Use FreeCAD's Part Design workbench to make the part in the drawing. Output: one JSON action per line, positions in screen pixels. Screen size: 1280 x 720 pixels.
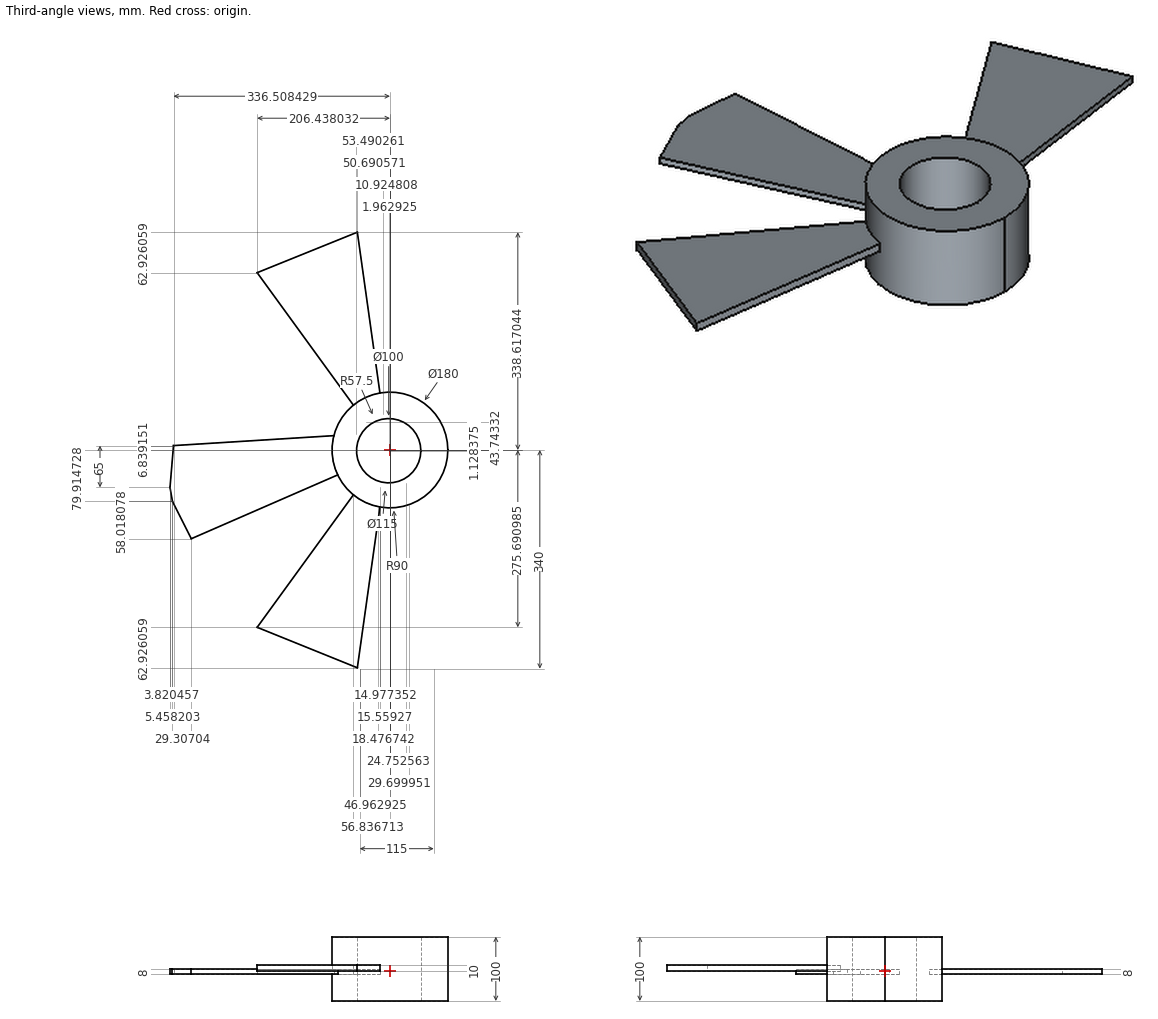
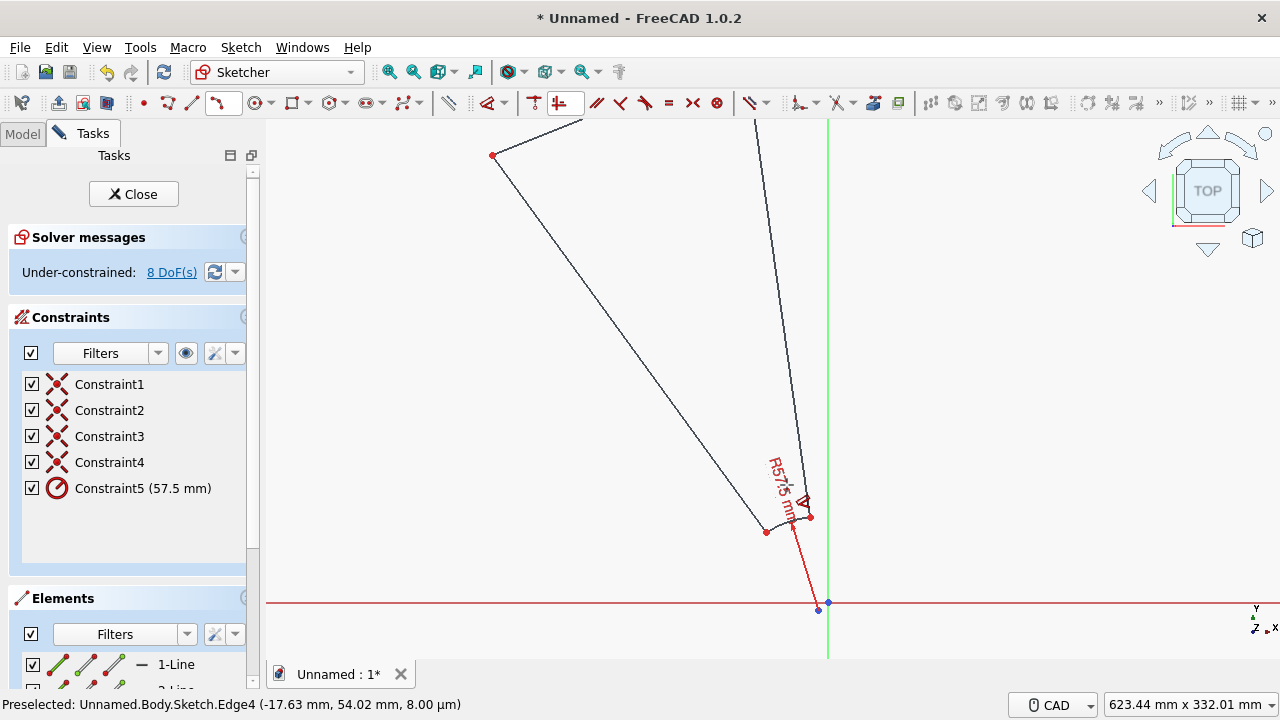
{"action": "left_click", "coordinate": [766, 533]}
{"action": "left_click", "coordinate": [862, 568]}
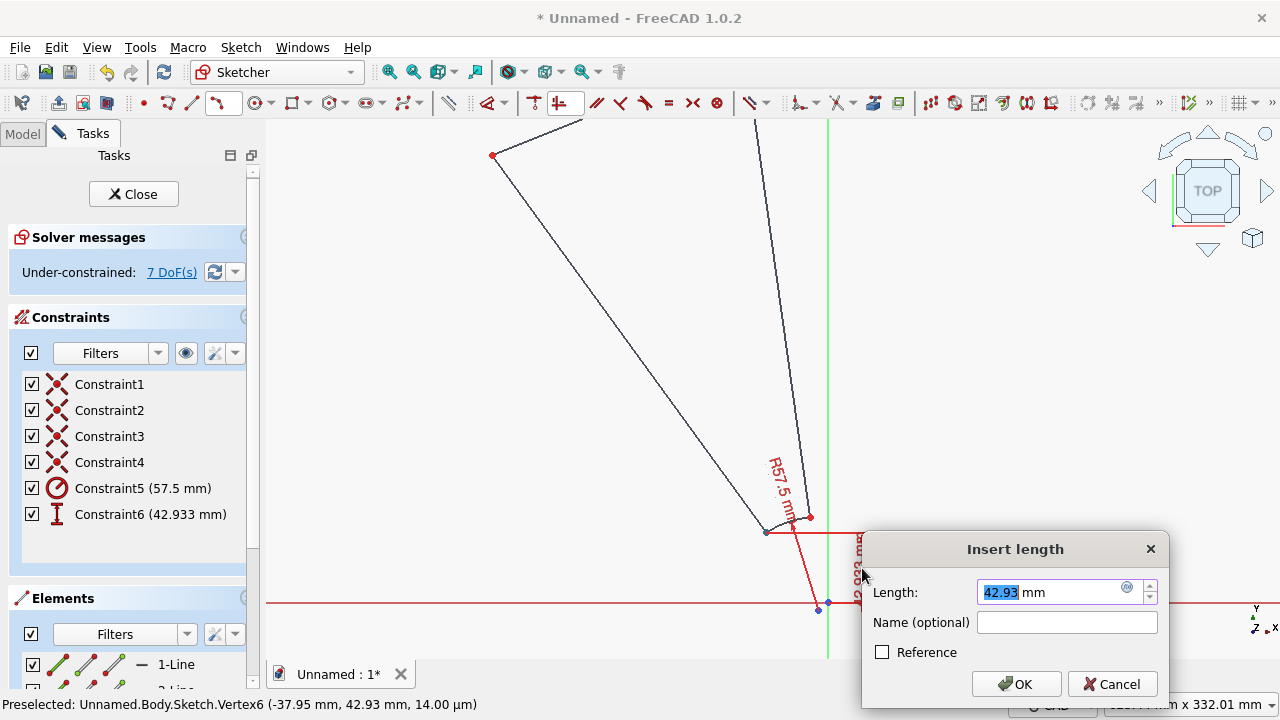
{"action": "type", "text": "43.74332"}
{"action": "key", "text": "Return"}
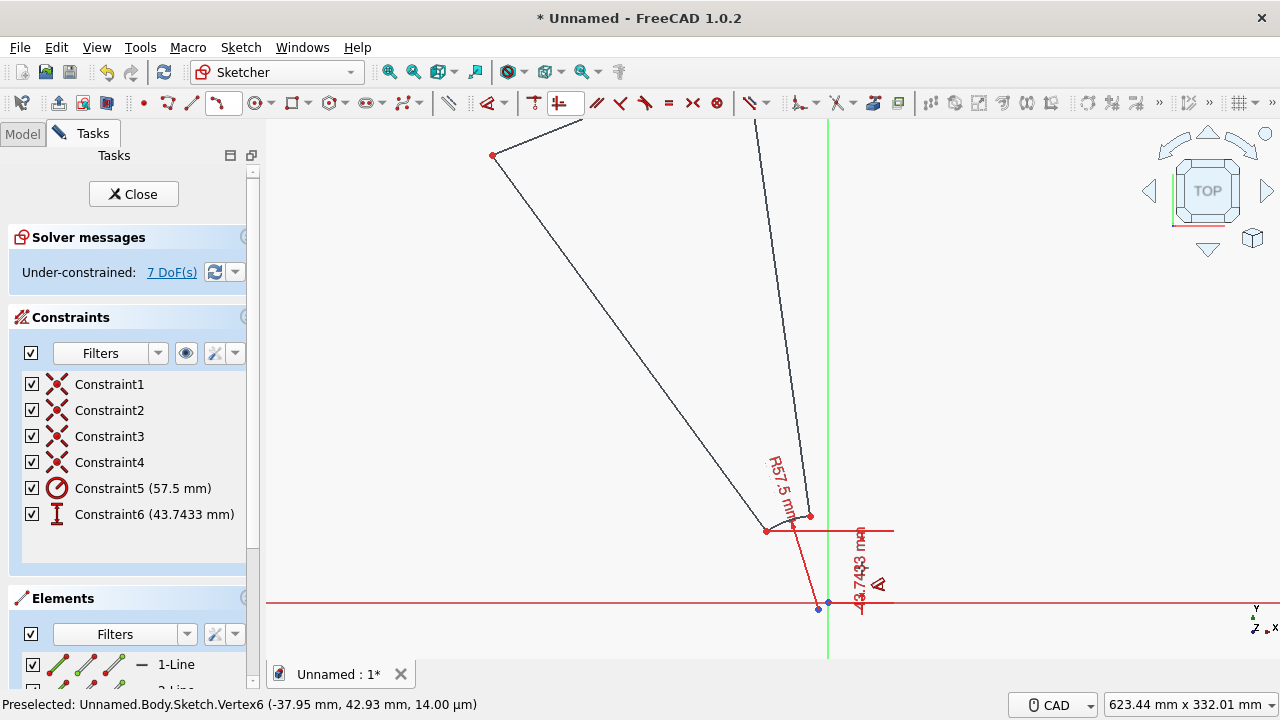
{"action": "scroll", "coordinate": [819, 609], "scroll_direction": "up", "scroll_amount": 13}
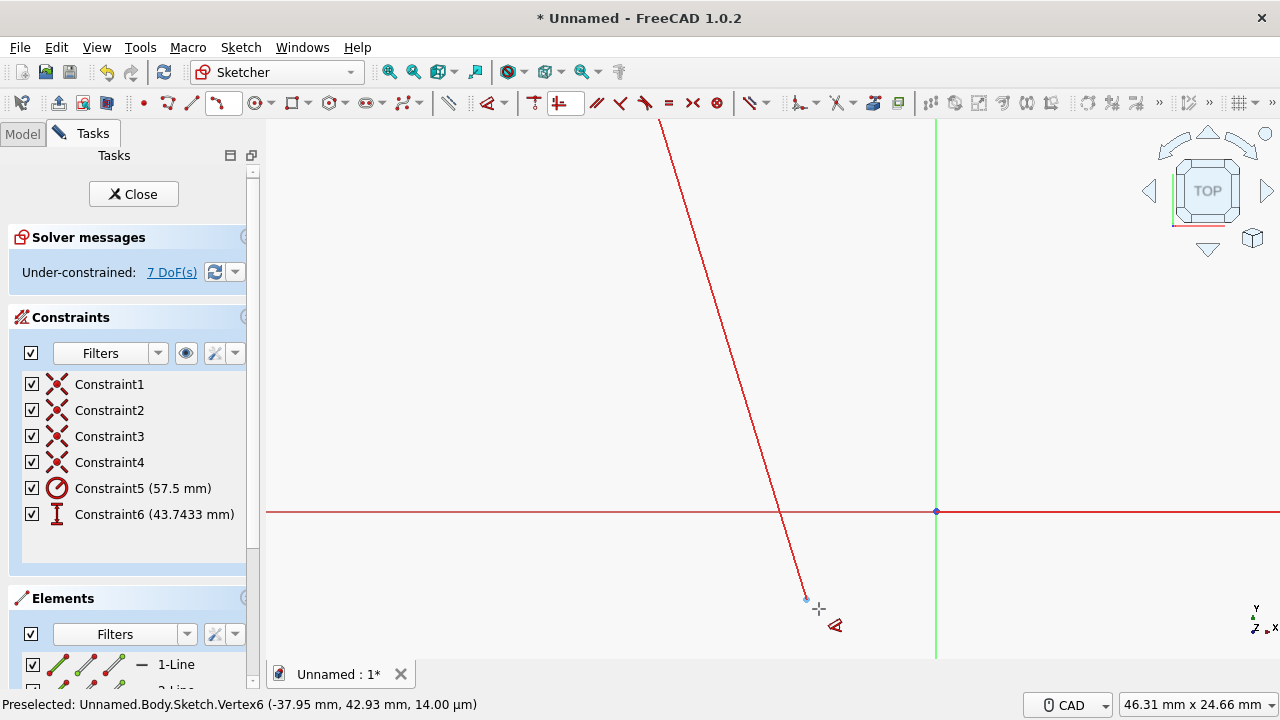
{"action": "left_click", "coordinate": [807, 599]}
{"action": "left_click", "coordinate": [871, 478]}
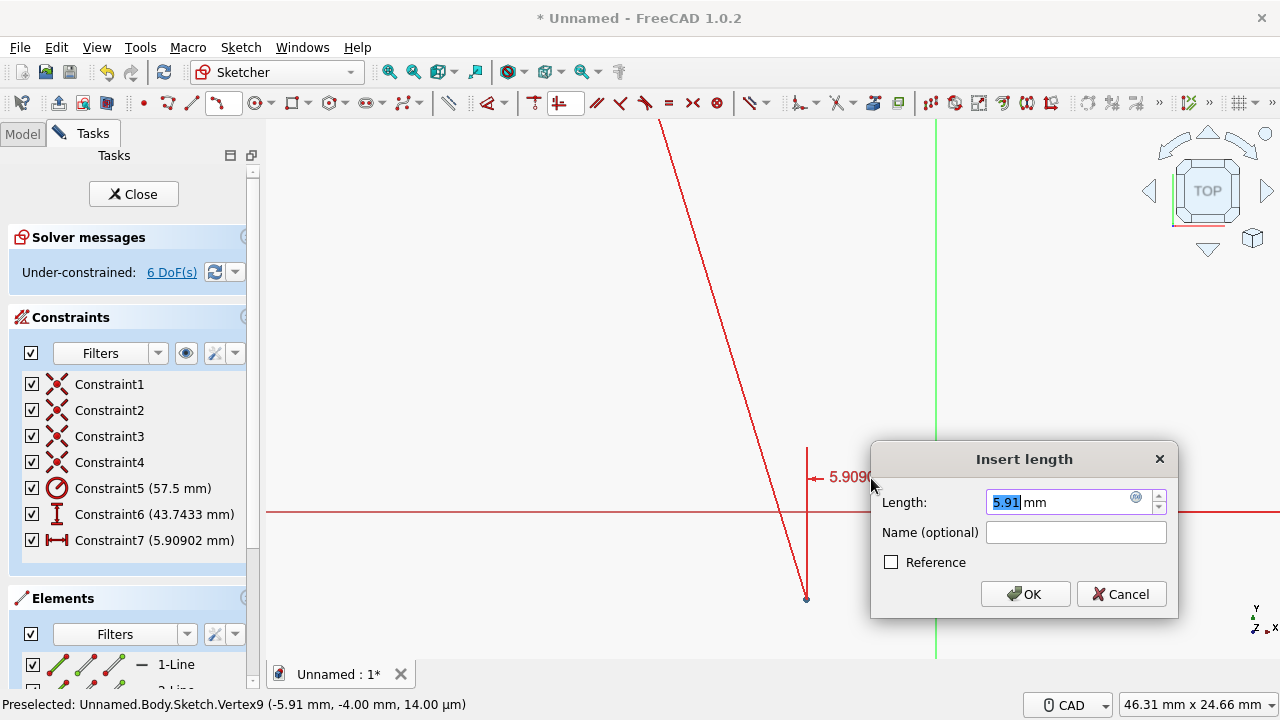
{"action": "type", "text": "1.962925"}
{"action": "key", "text": "Return"}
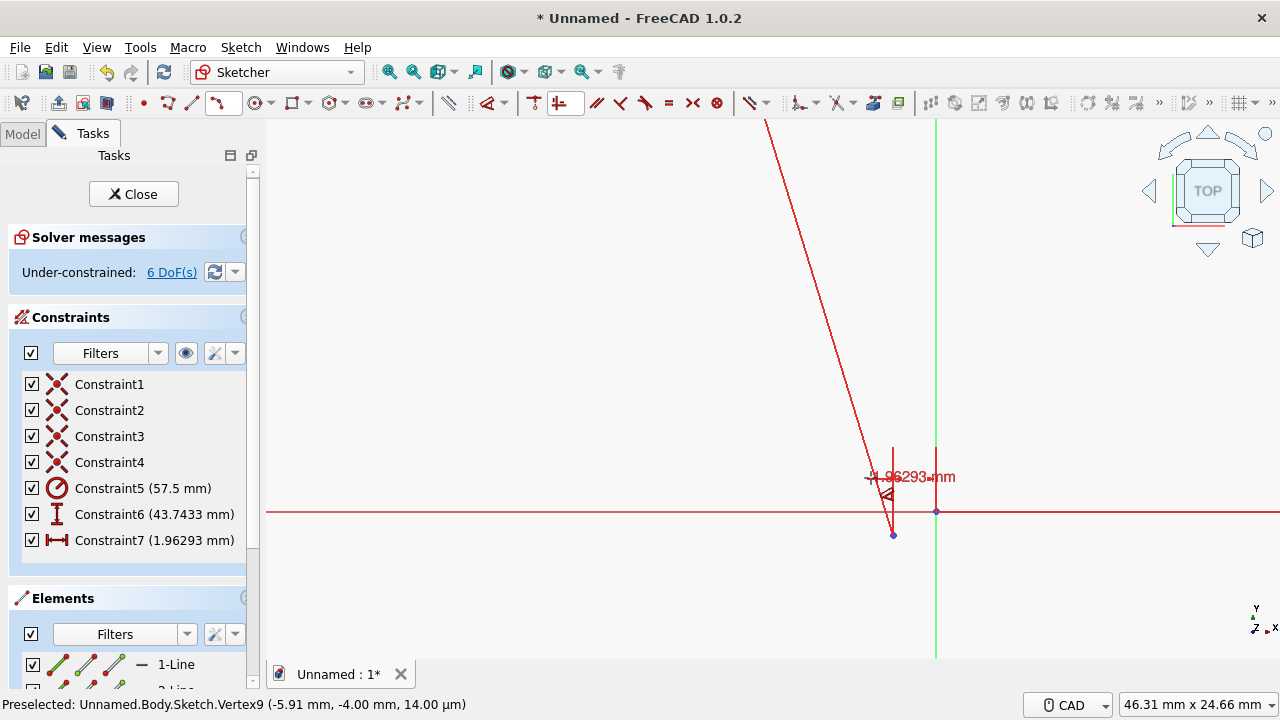
{"action": "scroll", "coordinate": [893, 536], "scroll_direction": "up", "scroll_amount": 3}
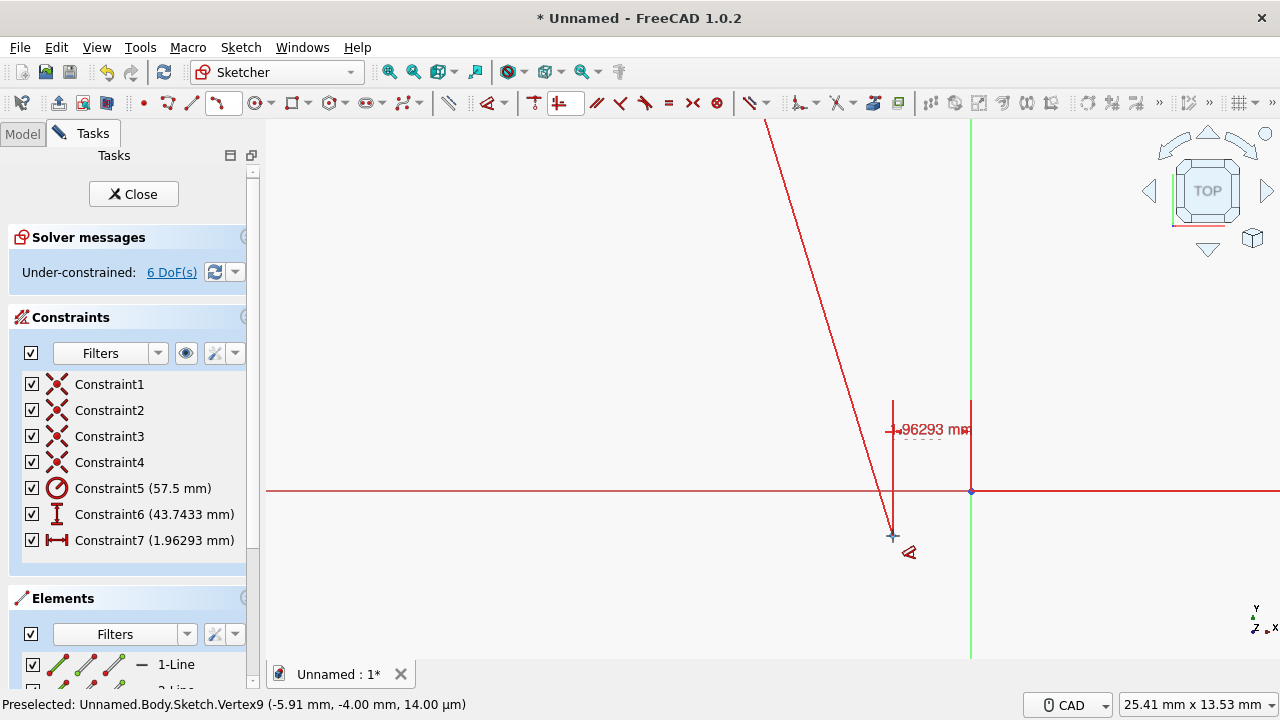
{"action": "left_click", "coordinate": [893, 535]}
{"action": "left_click", "coordinate": [1005, 513]}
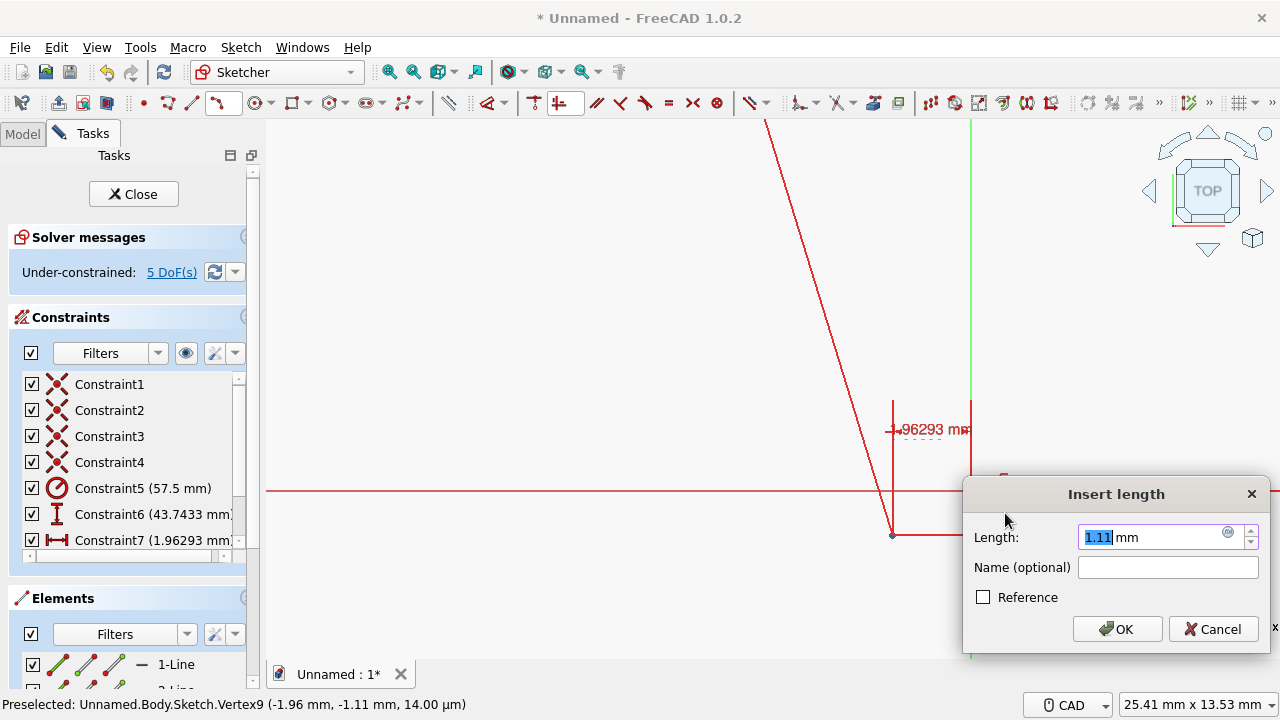
{"action": "type", "text": "1.128375"}
{"action": "key", "text": "Return"}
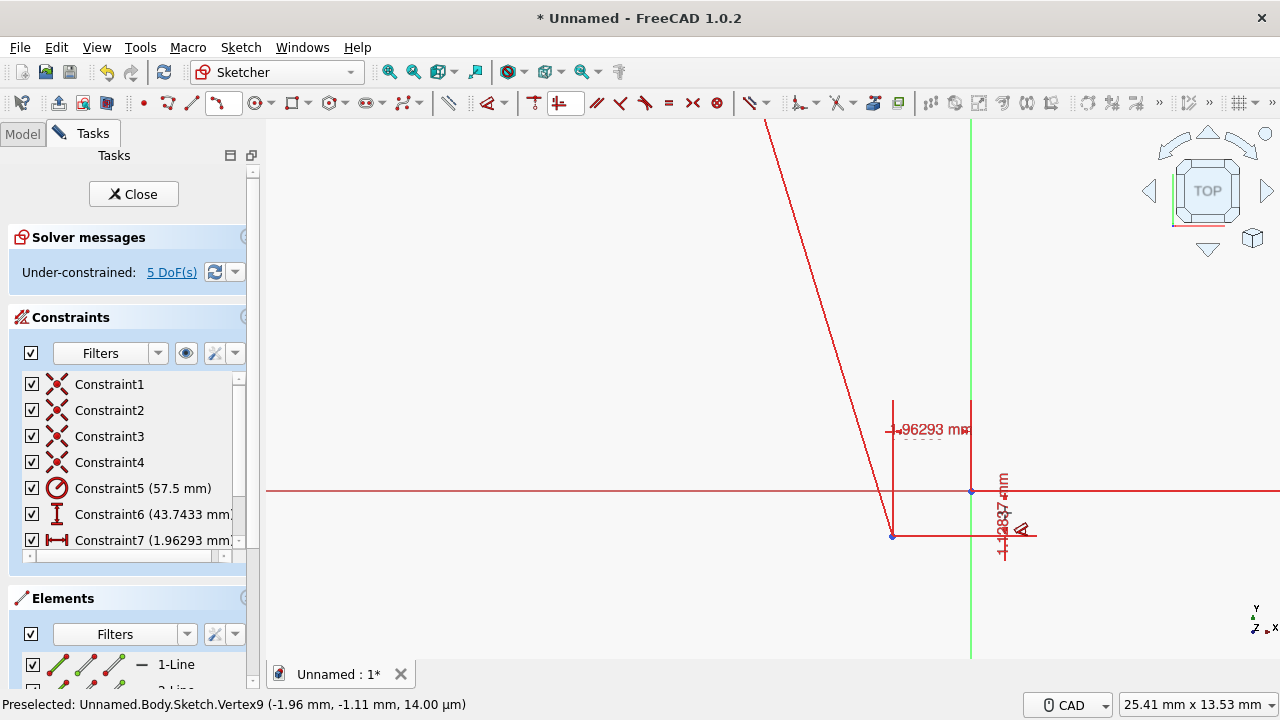
{"action": "scroll", "coordinate": [813, 576], "scroll_direction": "down", "scroll_amount": 18}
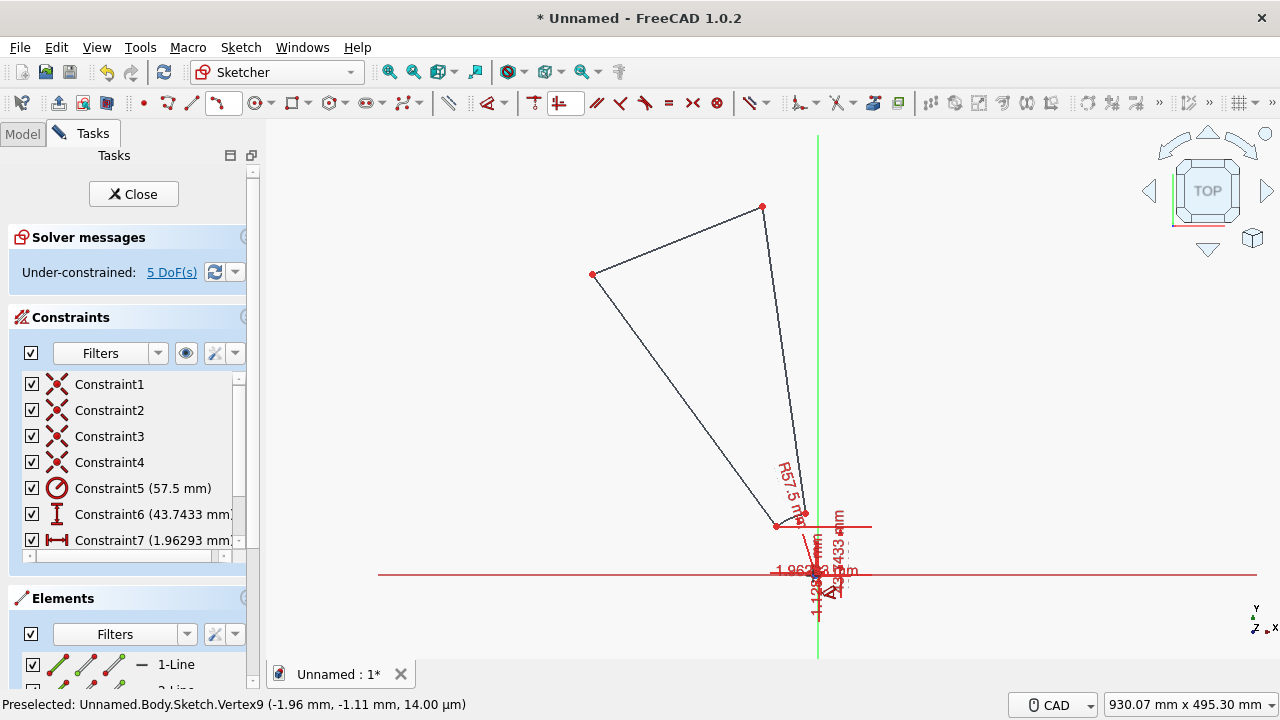
{"action": "scroll", "coordinate": [806, 514], "scroll_direction": "up", "scroll_amount": 7}